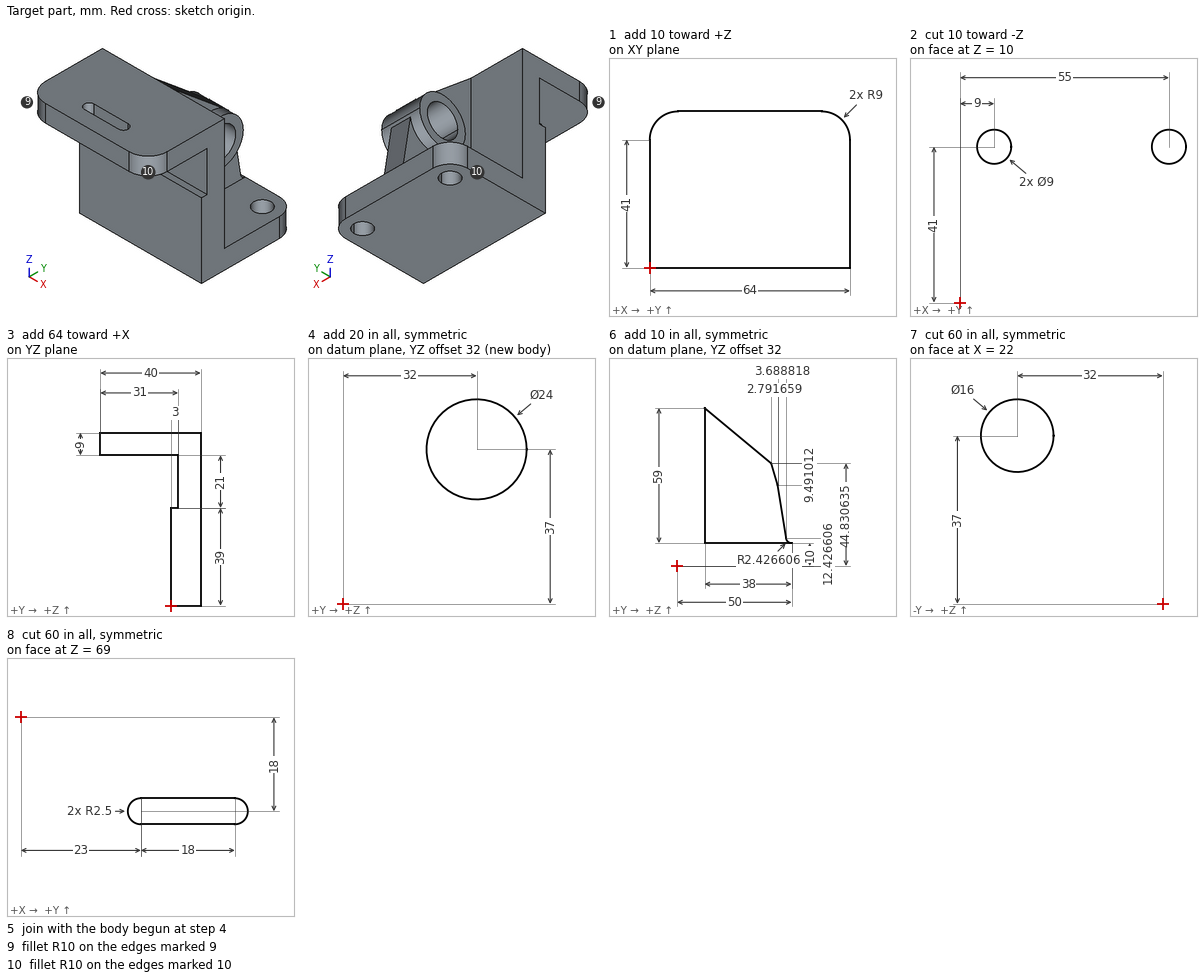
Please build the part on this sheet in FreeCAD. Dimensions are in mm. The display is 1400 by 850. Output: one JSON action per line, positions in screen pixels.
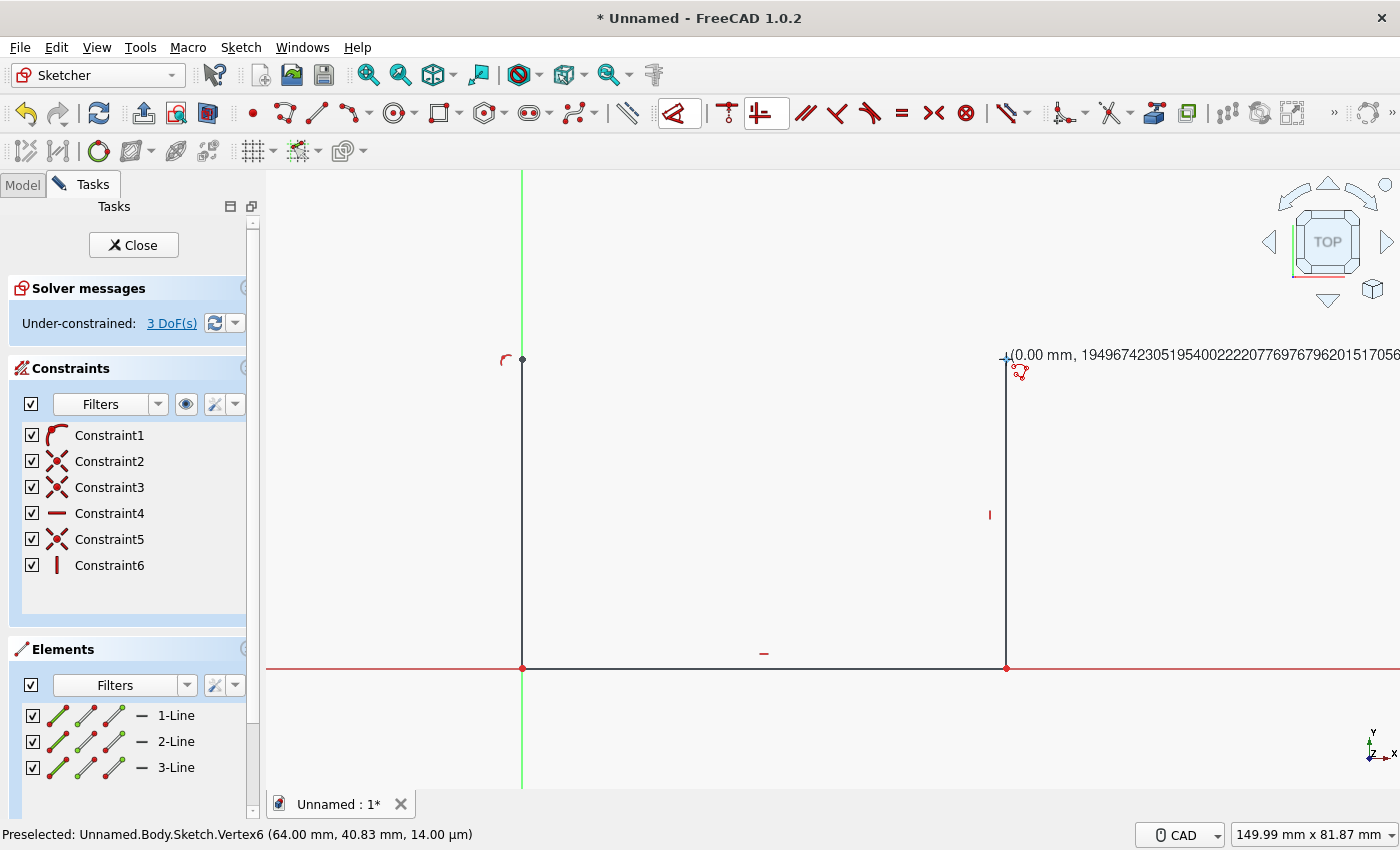
{"action": "left_click", "coordinate": [318, 114]}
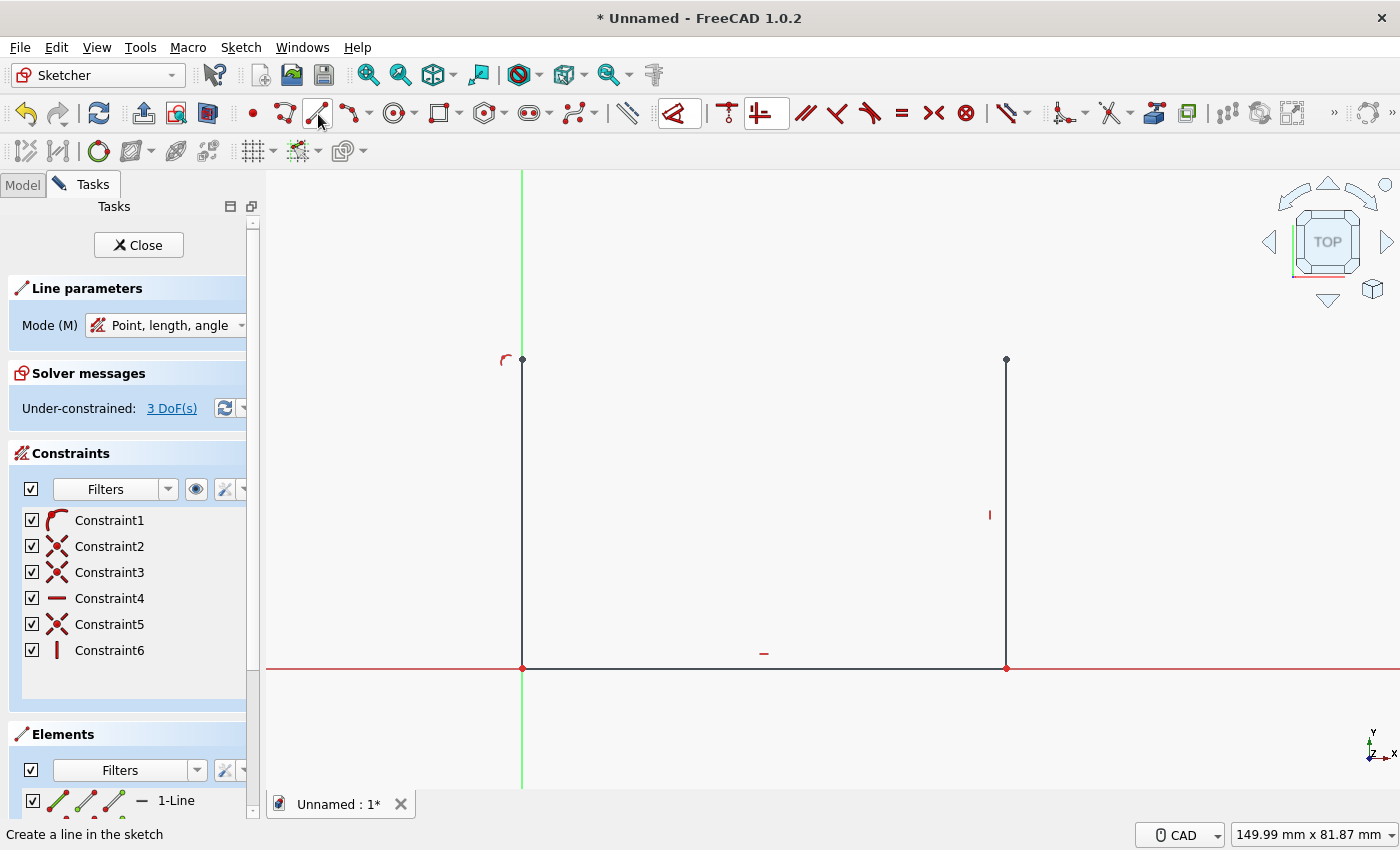
{"action": "left_click", "coordinate": [938, 291]}
{"action": "left_click", "coordinate": [590, 291]}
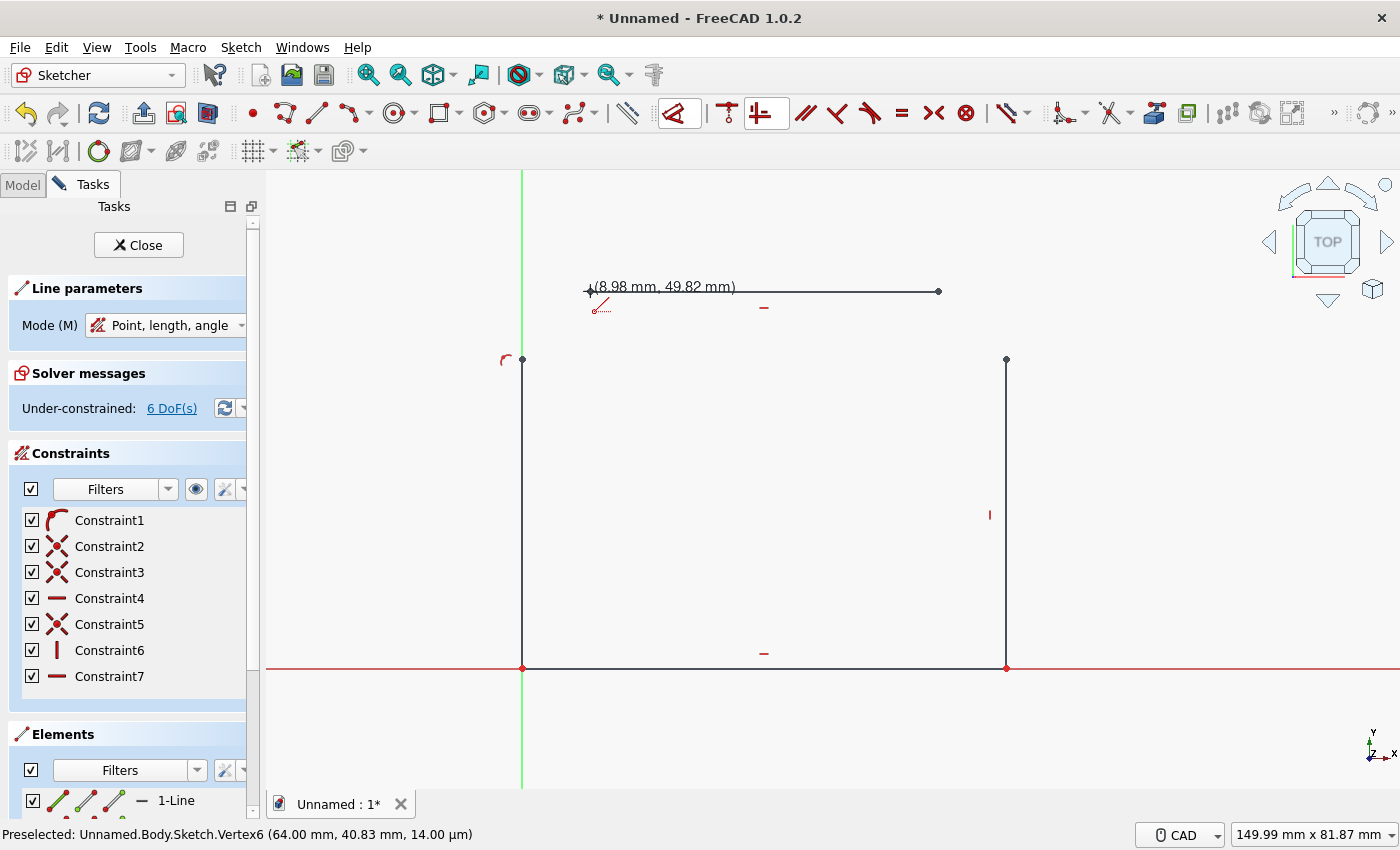
{"action": "left_click", "coordinate": [350, 114]}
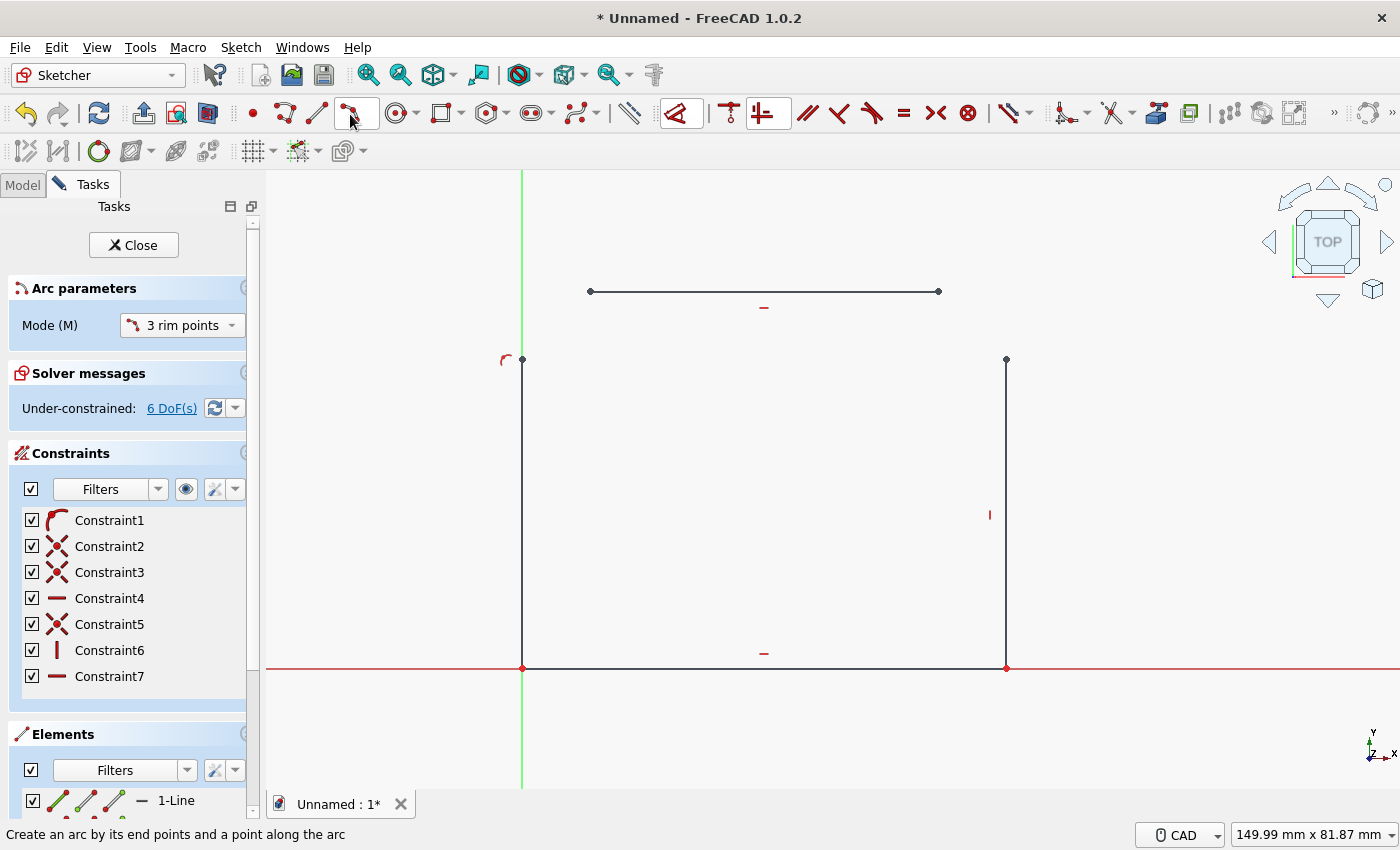
{"action": "left_click", "coordinate": [1006, 360]}
{"action": "left_click", "coordinate": [938, 292]}
{"action": "left_click", "coordinate": [986, 311]}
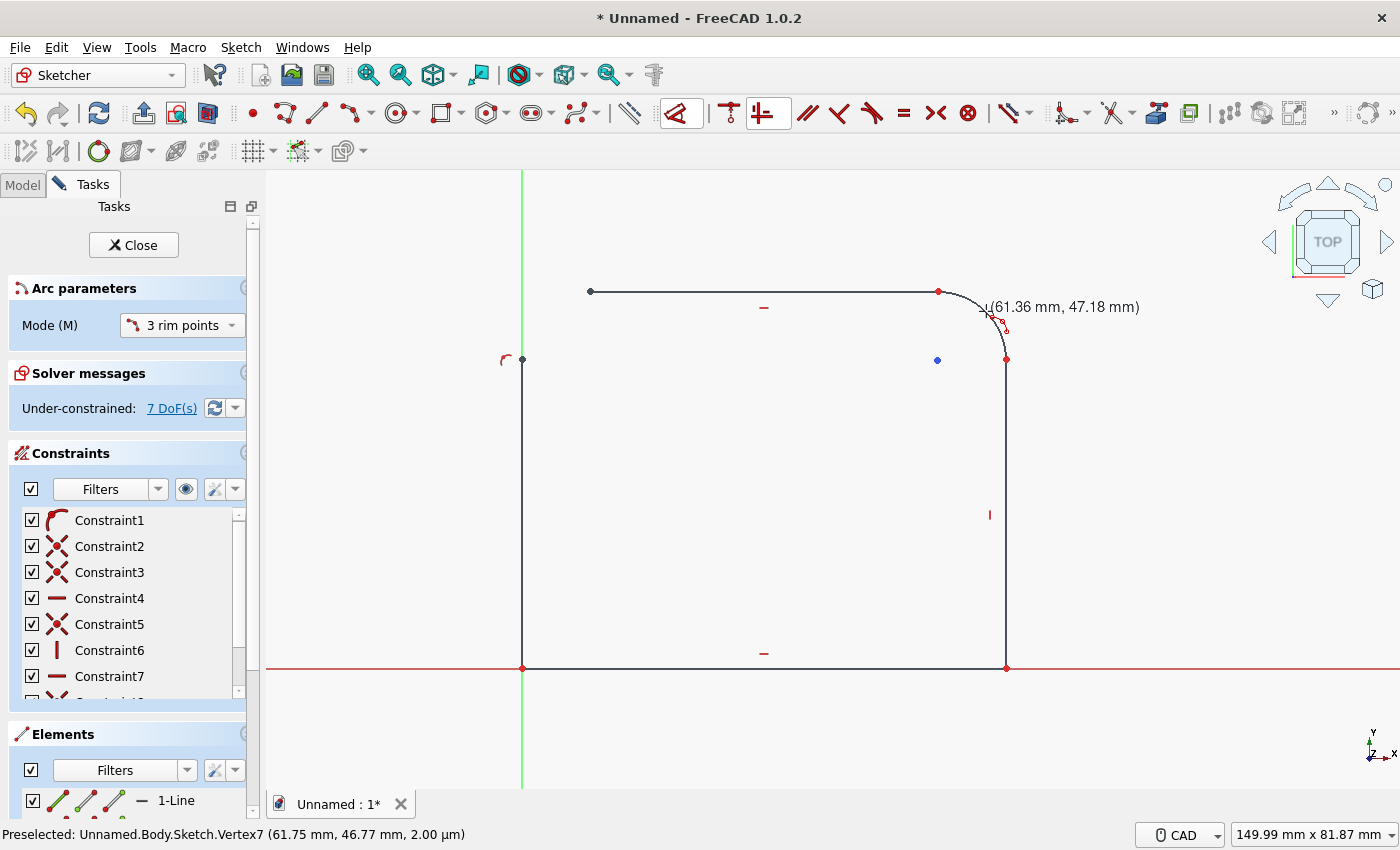
{"action": "left_click", "coordinate": [590, 292]}
{"action": "left_click", "coordinate": [522, 360]}
{"action": "left_click", "coordinate": [542, 311]}
{"action": "key", "text": "Escape"}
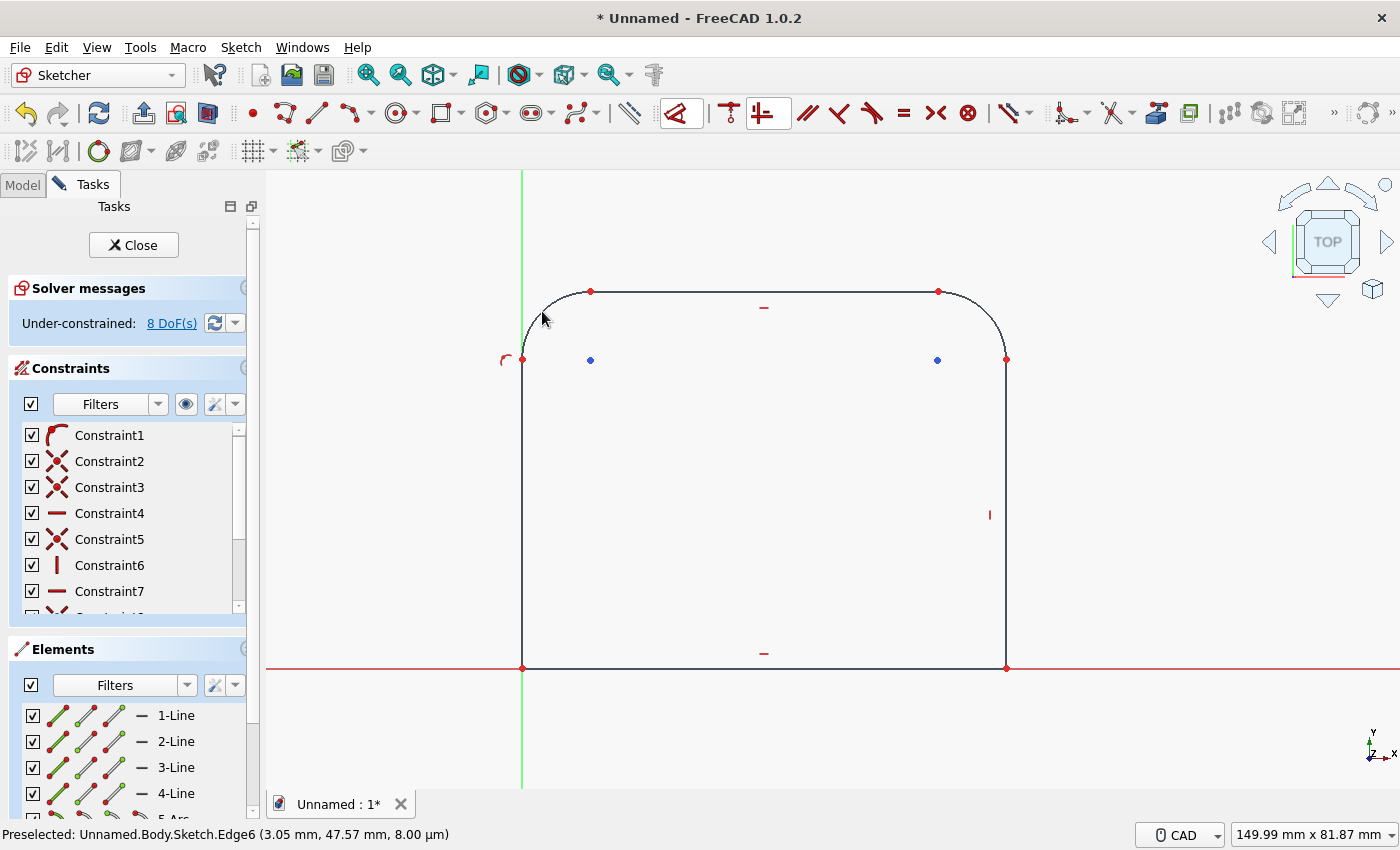
{"action": "left_click", "coordinate": [522, 453]}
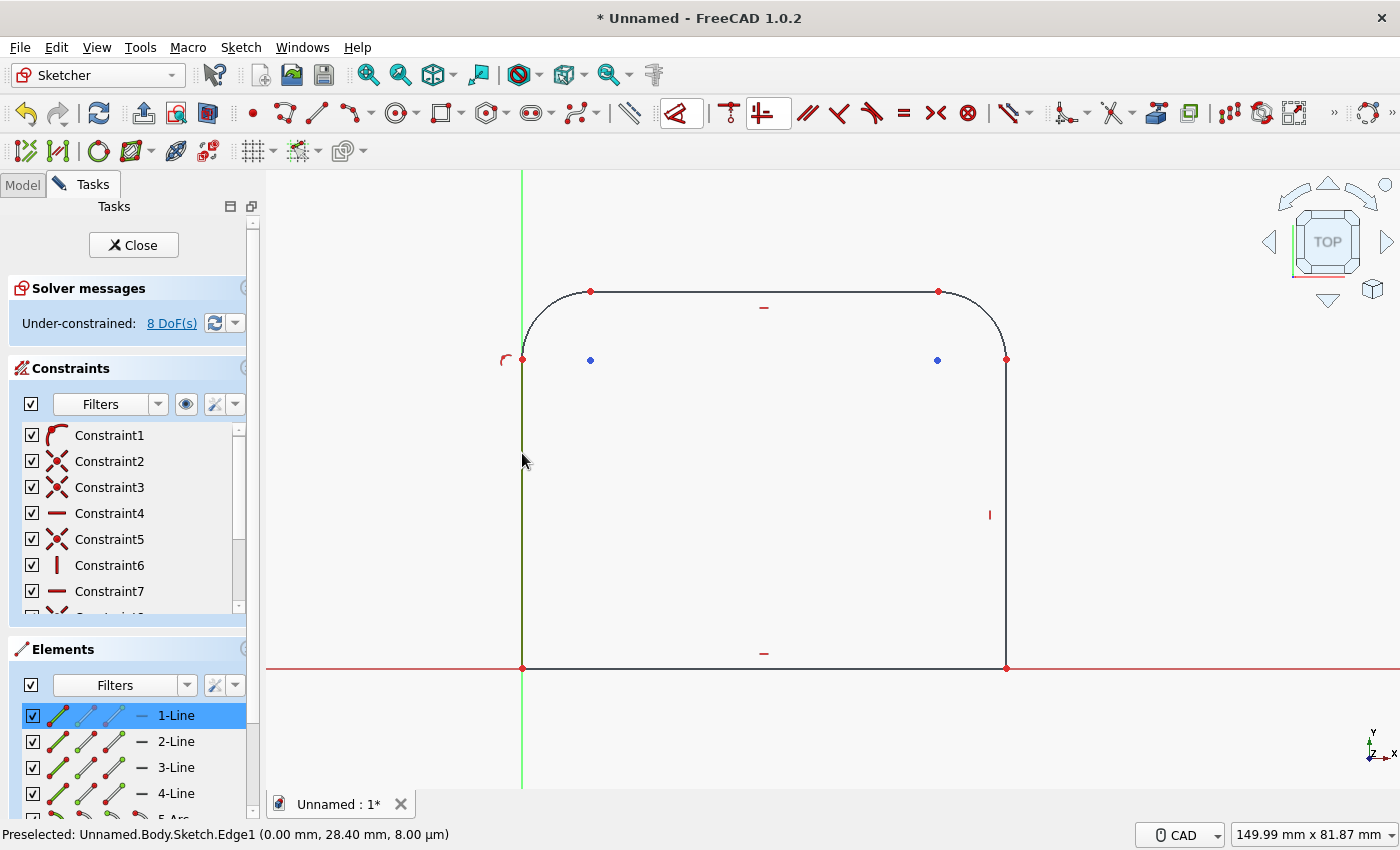
{"action": "left_click", "coordinate": [559, 299]}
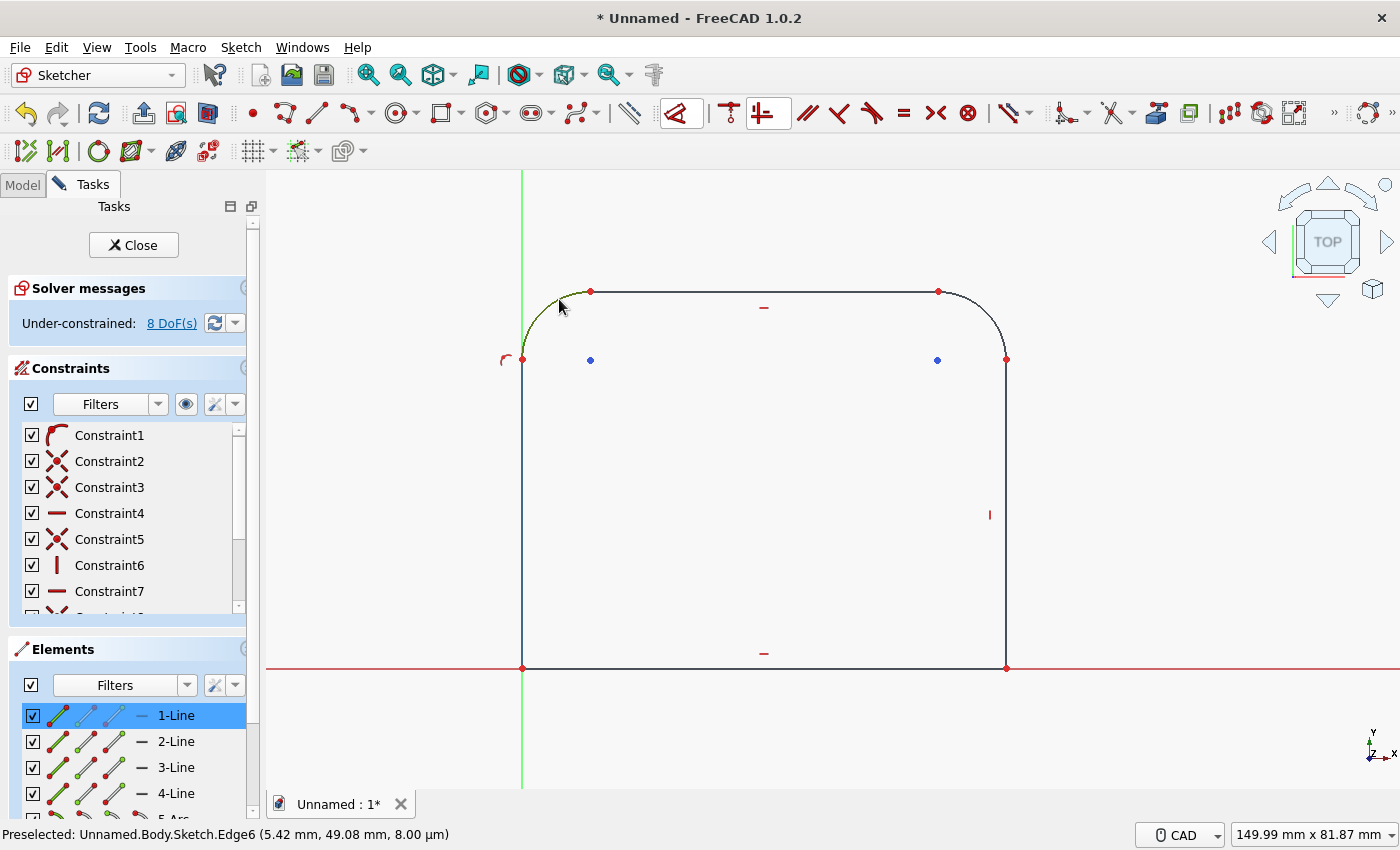
{"action": "left_click", "coordinate": [872, 114]}